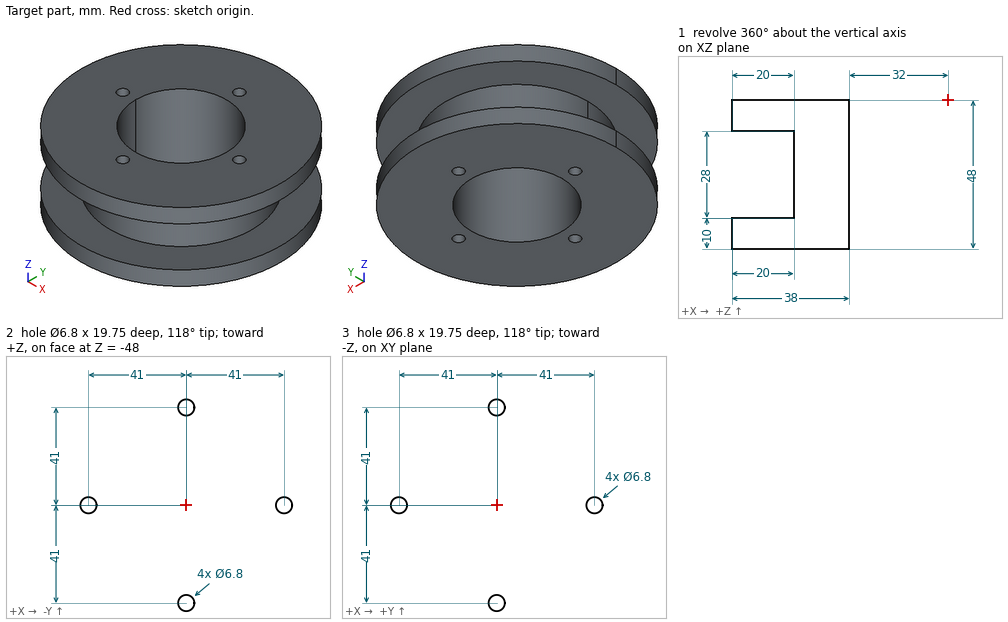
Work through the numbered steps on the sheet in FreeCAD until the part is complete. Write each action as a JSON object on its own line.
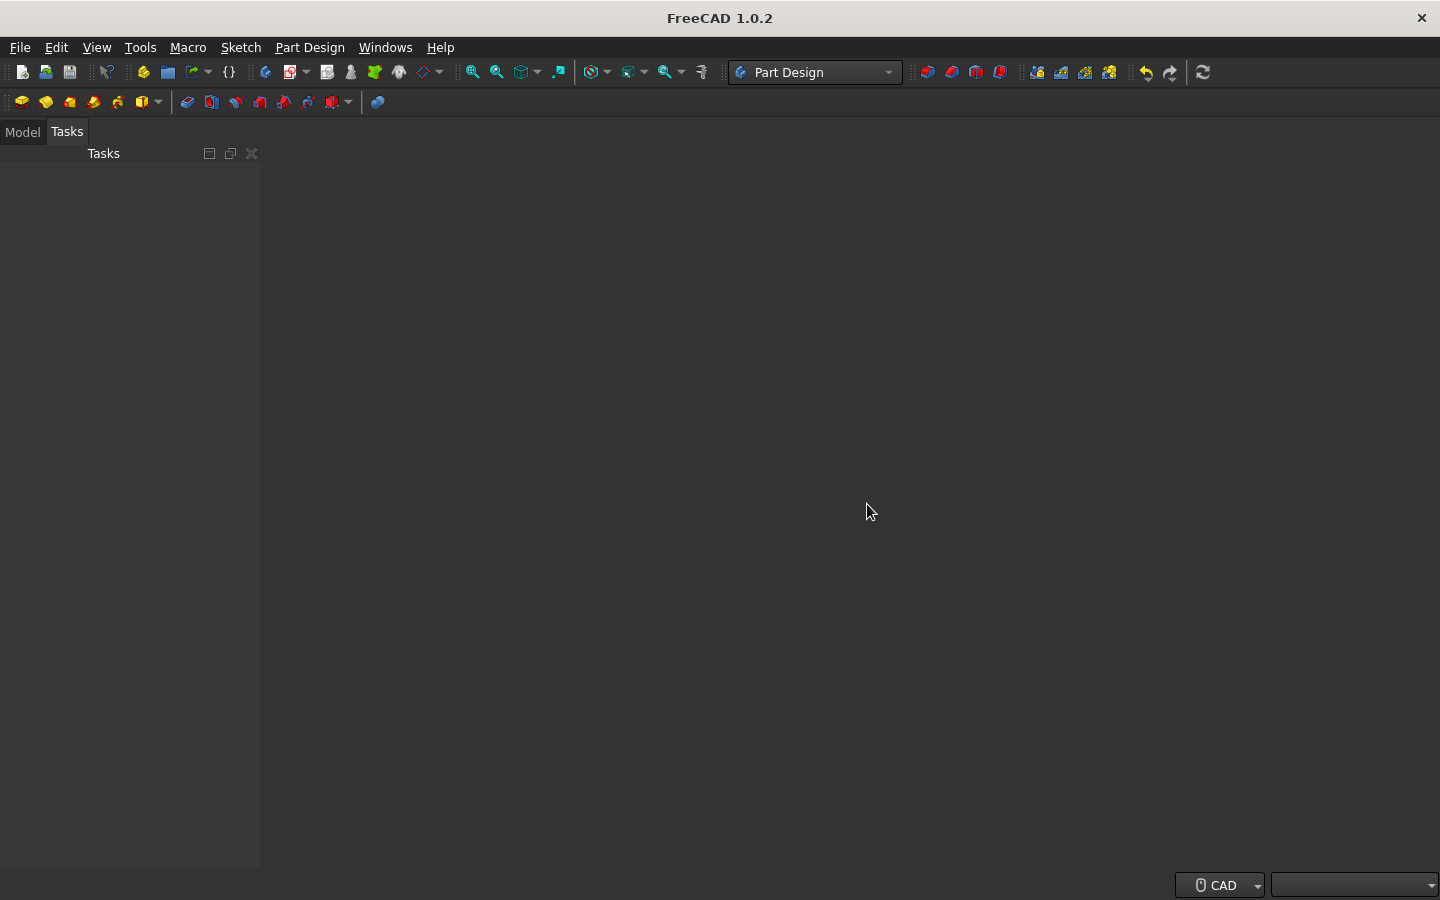
{"action": "left_click", "coordinate": [22, 72]}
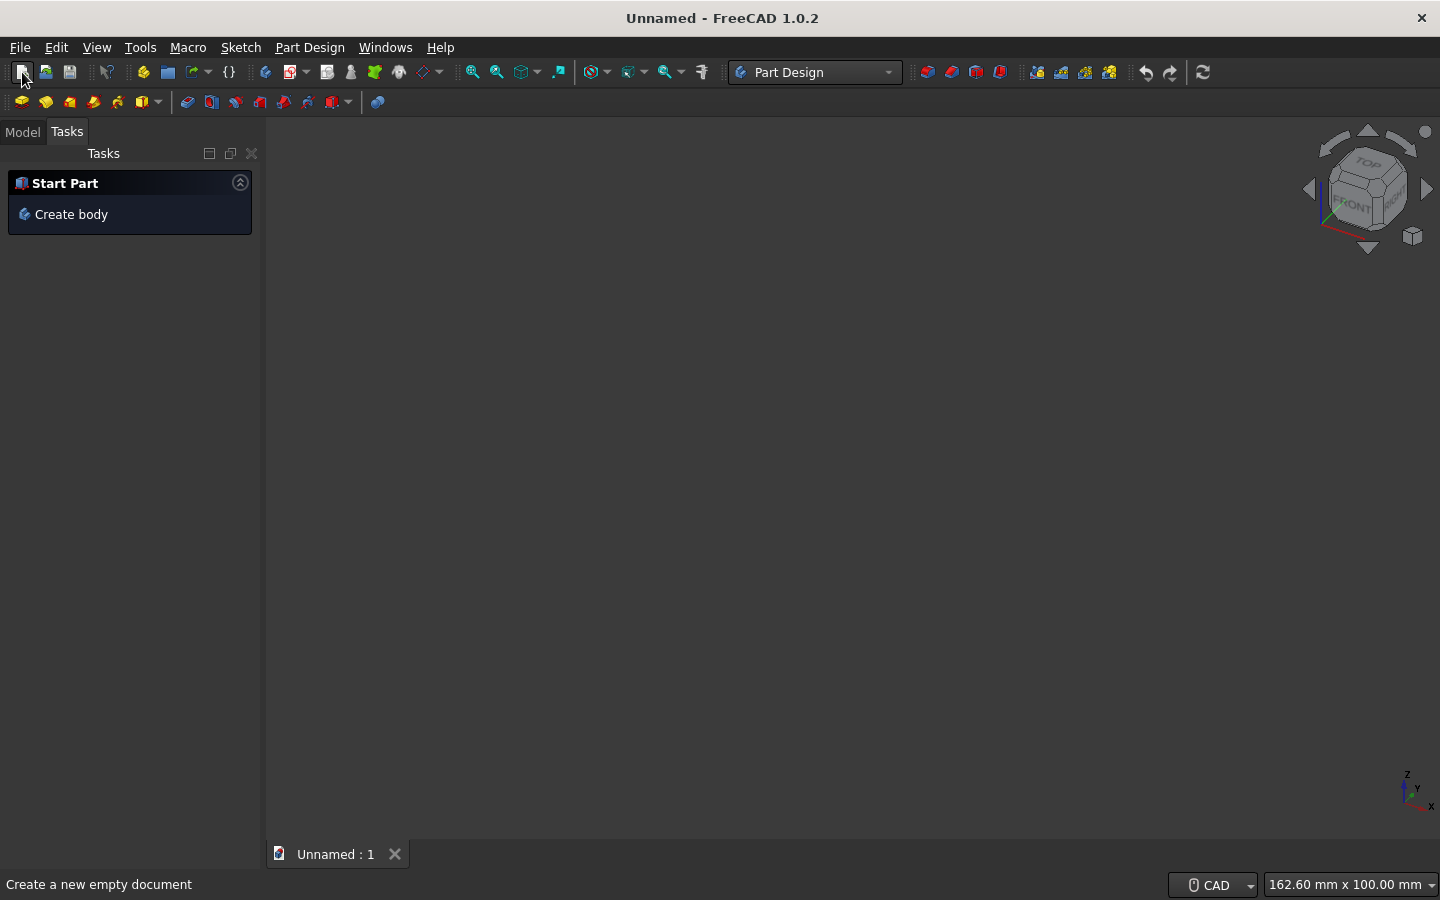
{"action": "left_click", "coordinate": [290, 72]}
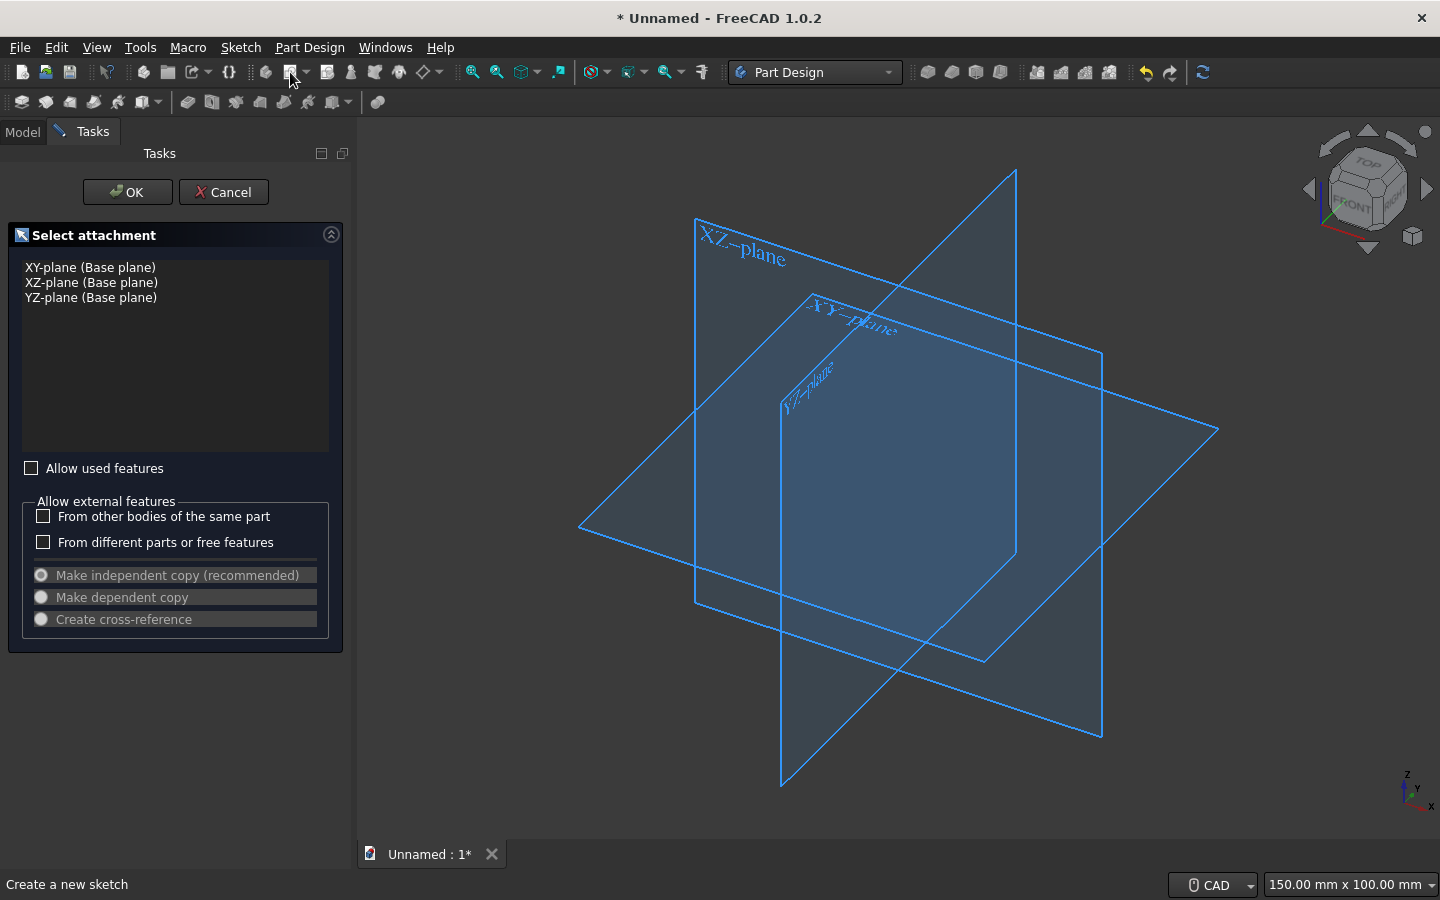
{"action": "left_click", "coordinate": [82, 282]}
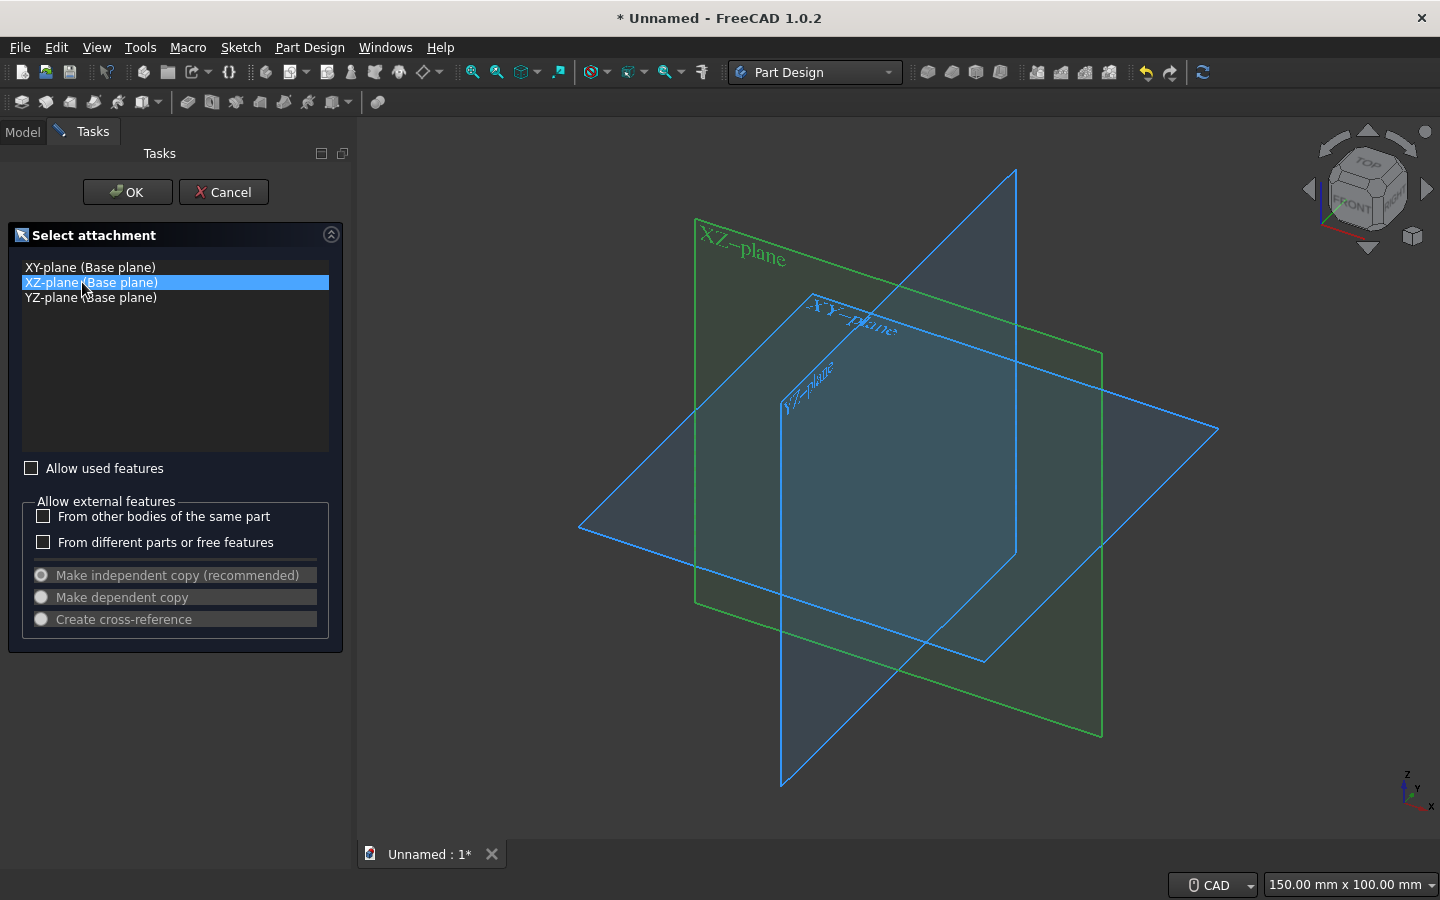
{"action": "left_click", "coordinate": [128, 192]}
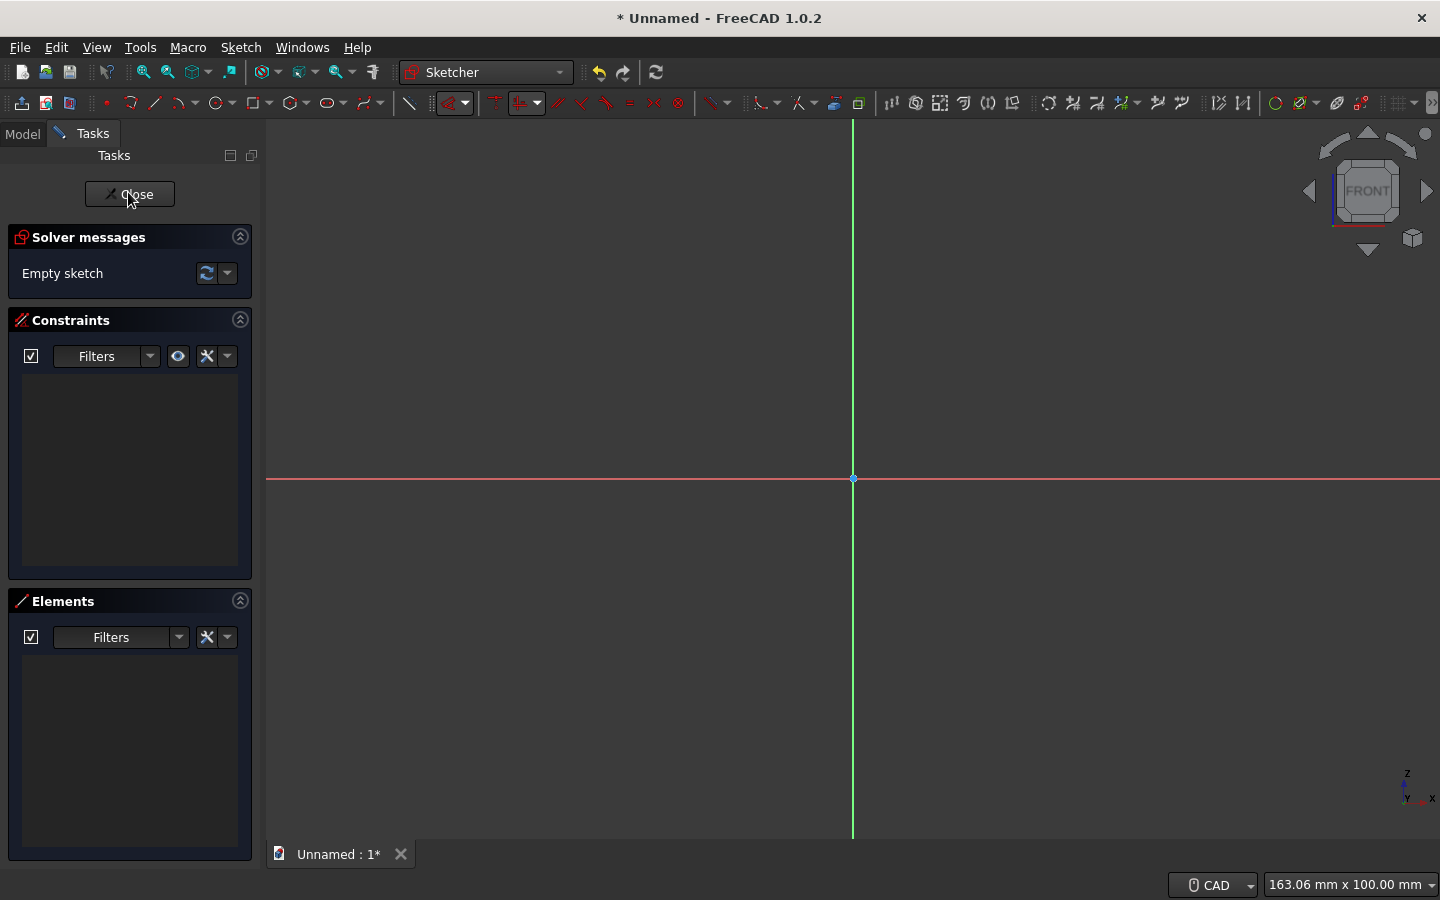
{"action": "scroll", "coordinate": [1275, 147], "scroll_direction": "down", "scroll_amount": 1}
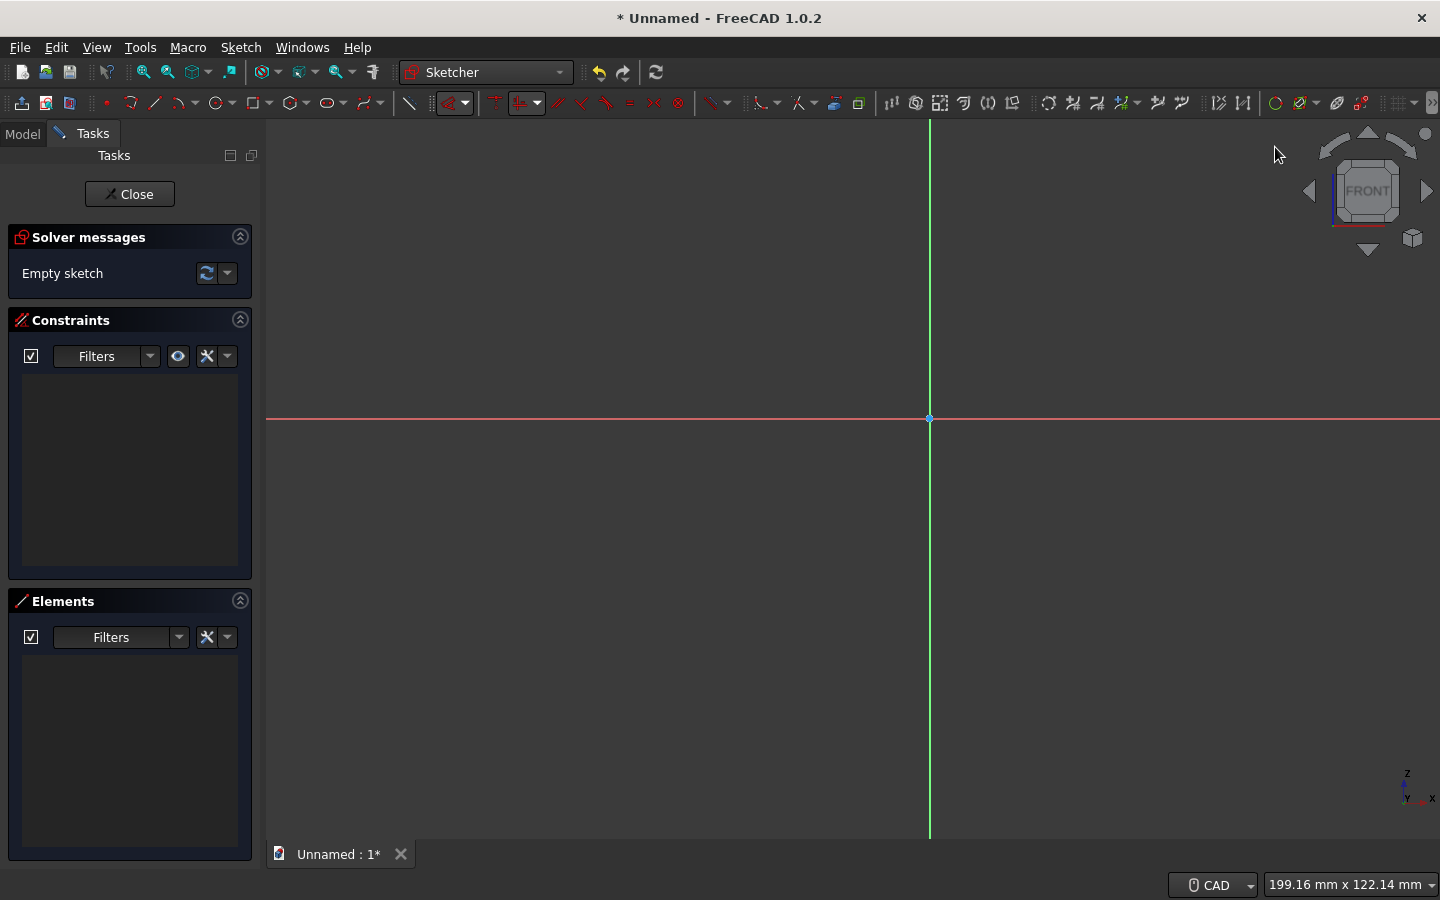
{"action": "scroll", "coordinate": [649, 659], "scroll_direction": "up", "scroll_amount": 3}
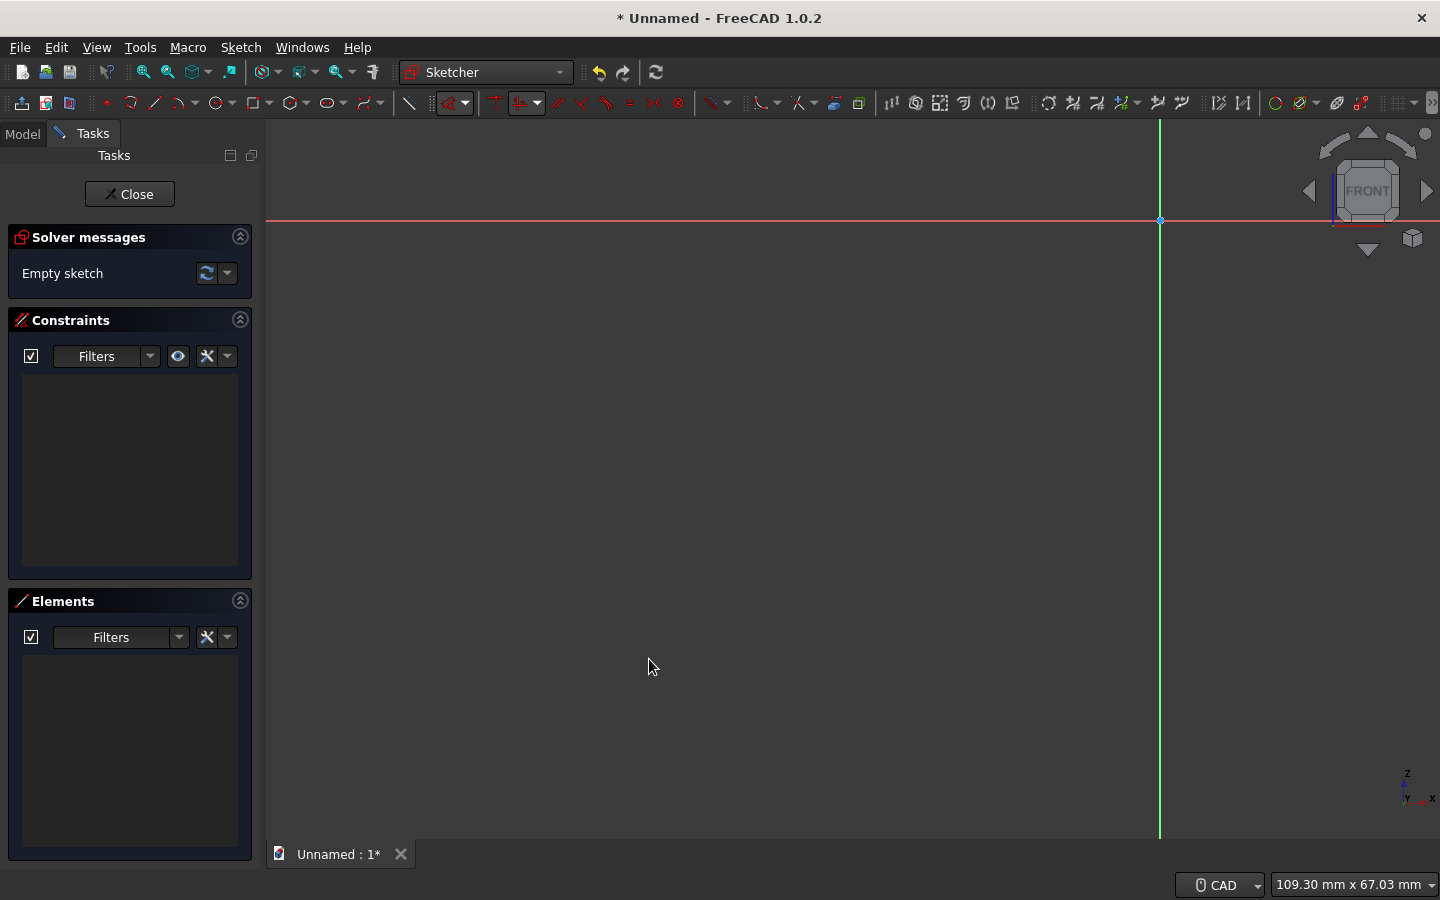
{"action": "left_click", "coordinate": [132, 104]}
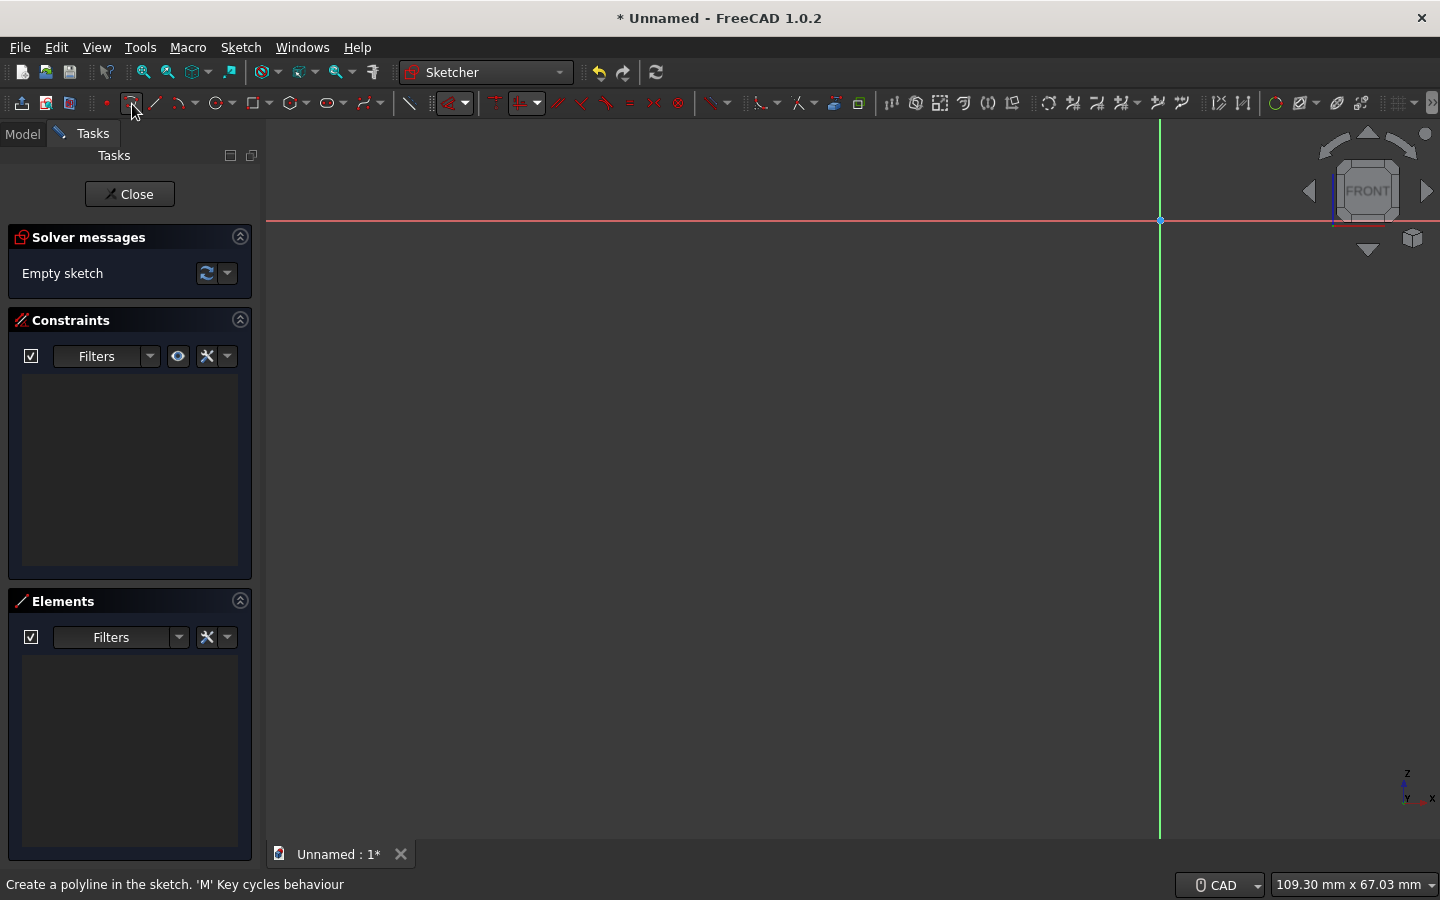
{"action": "left_click", "coordinate": [816, 221]}
{"action": "left_click", "coordinate": [816, 736]}
{"action": "left_click", "coordinate": [408, 736]}
{"action": "left_click", "coordinate": [408, 629]}
{"action": "left_click", "coordinate": [623, 629]}
{"action": "left_click", "coordinate": [623, 328]}
{"action": "left_click", "coordinate": [408, 328]}
{"action": "left_click", "coordinate": [408, 230]}
{"action": "left_click", "coordinate": [816, 221]}
{"action": "key", "text": "Escape"}
{"action": "key", "text": "Escape"}